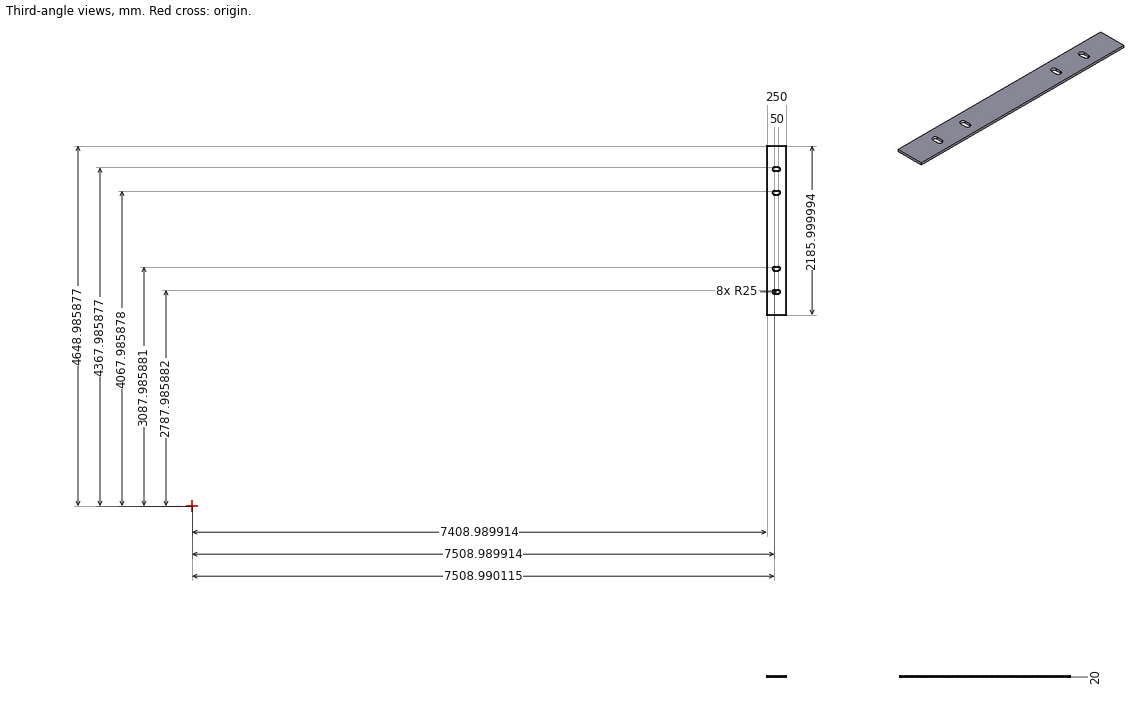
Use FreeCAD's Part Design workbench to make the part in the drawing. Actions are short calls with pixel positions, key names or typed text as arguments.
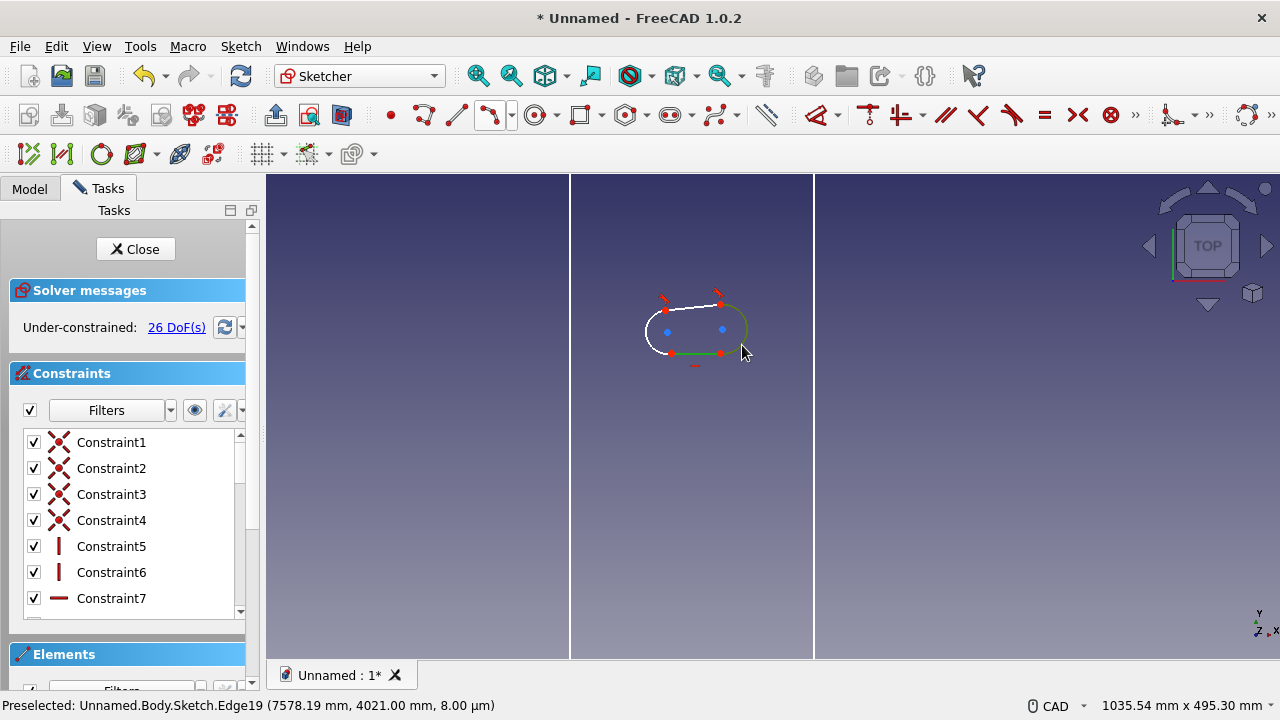
key(t)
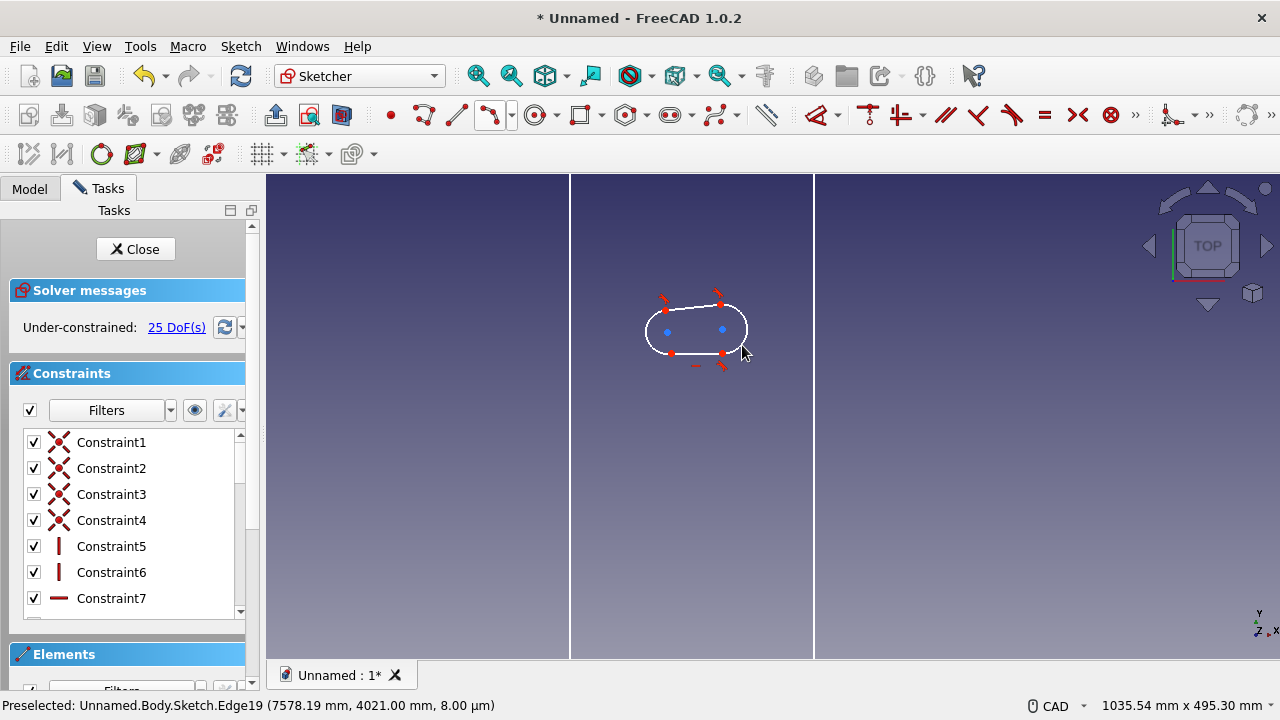
click(707, 354)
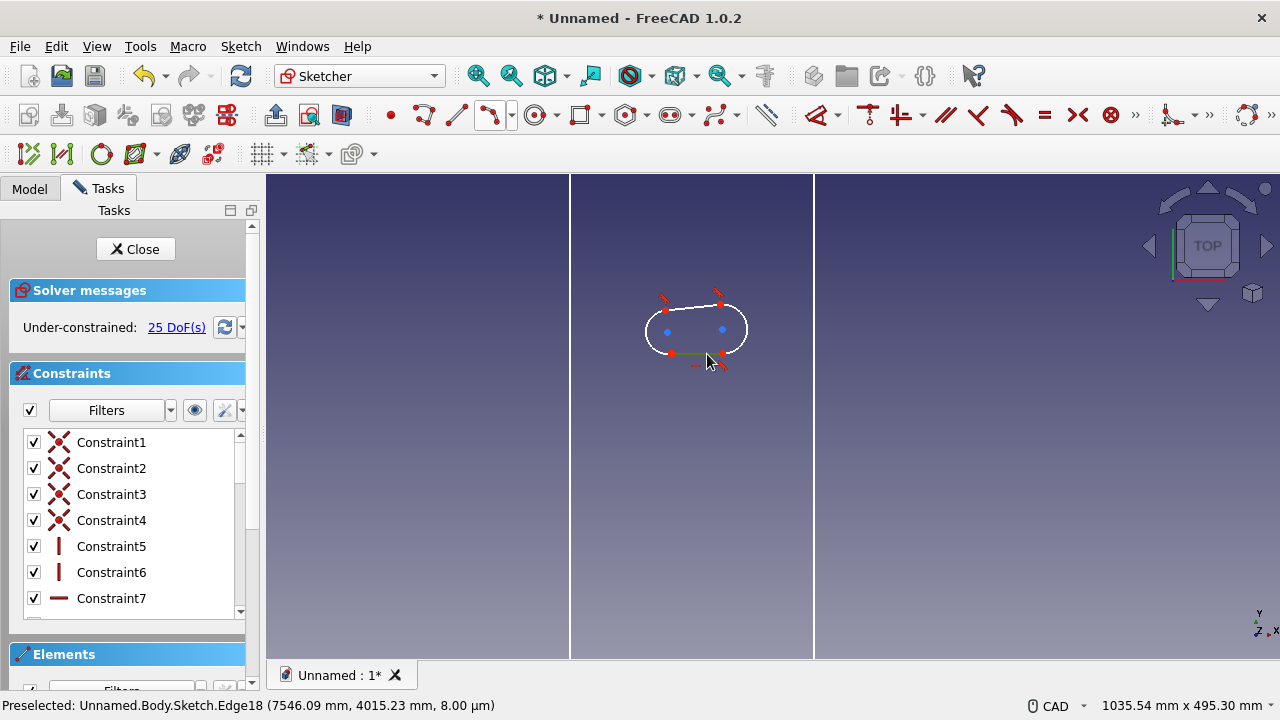
click(649, 322)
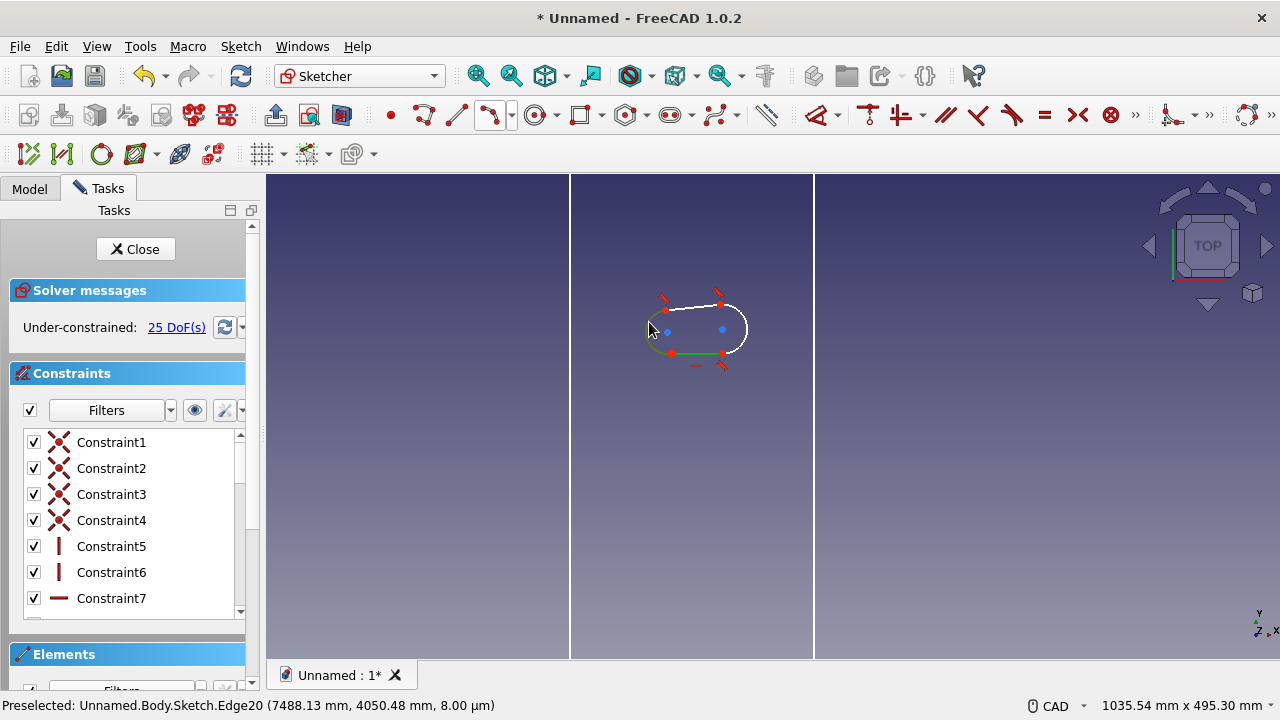
click(1012, 116)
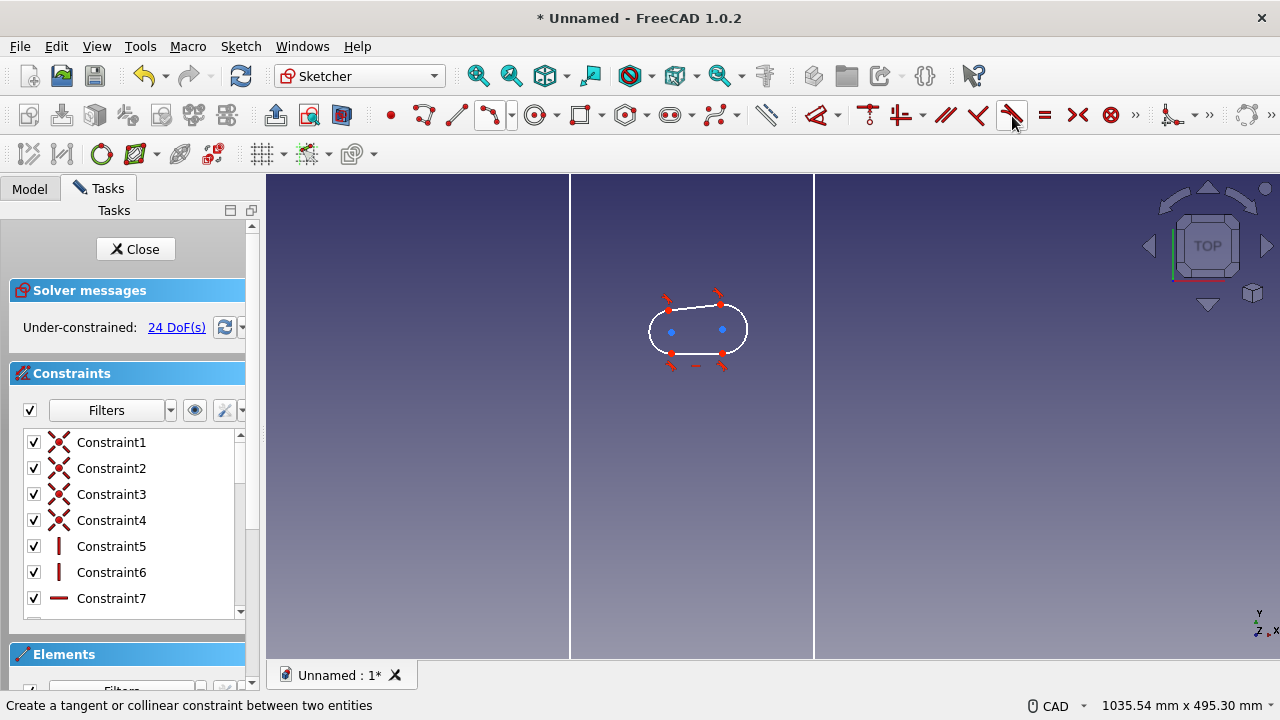
scroll(706, 356, down, 10)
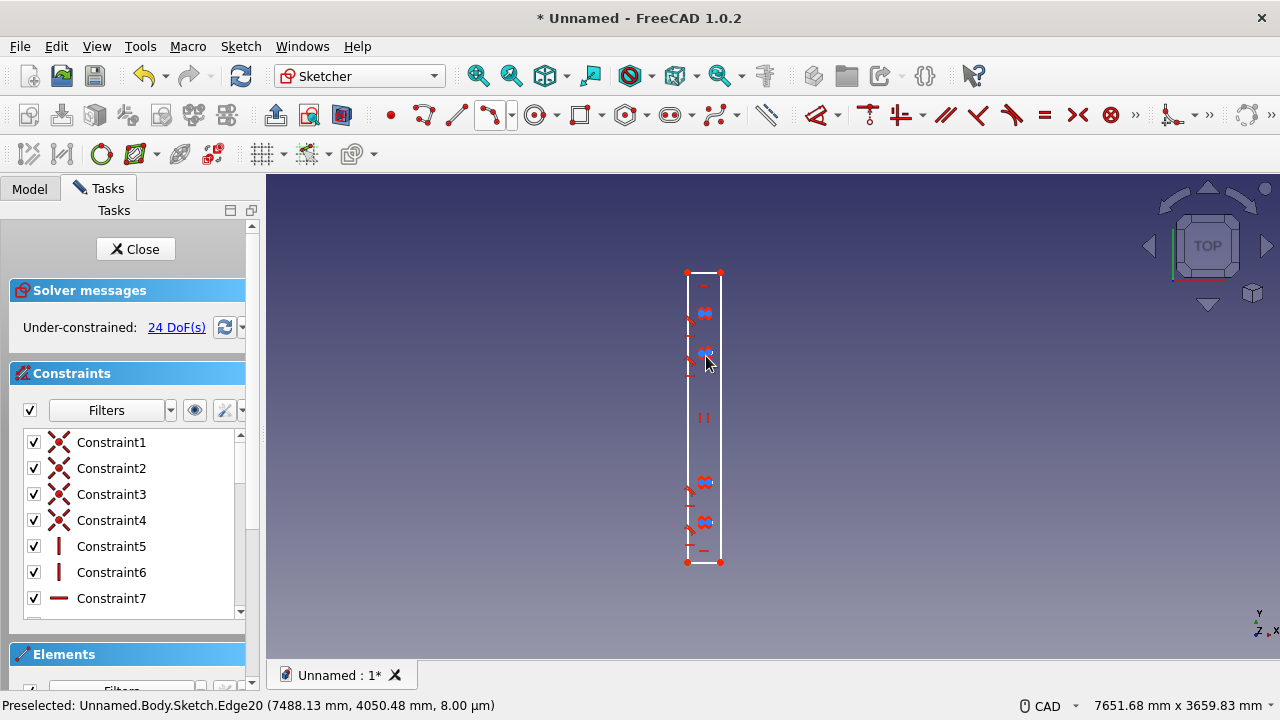
scroll(704, 520, up, 10)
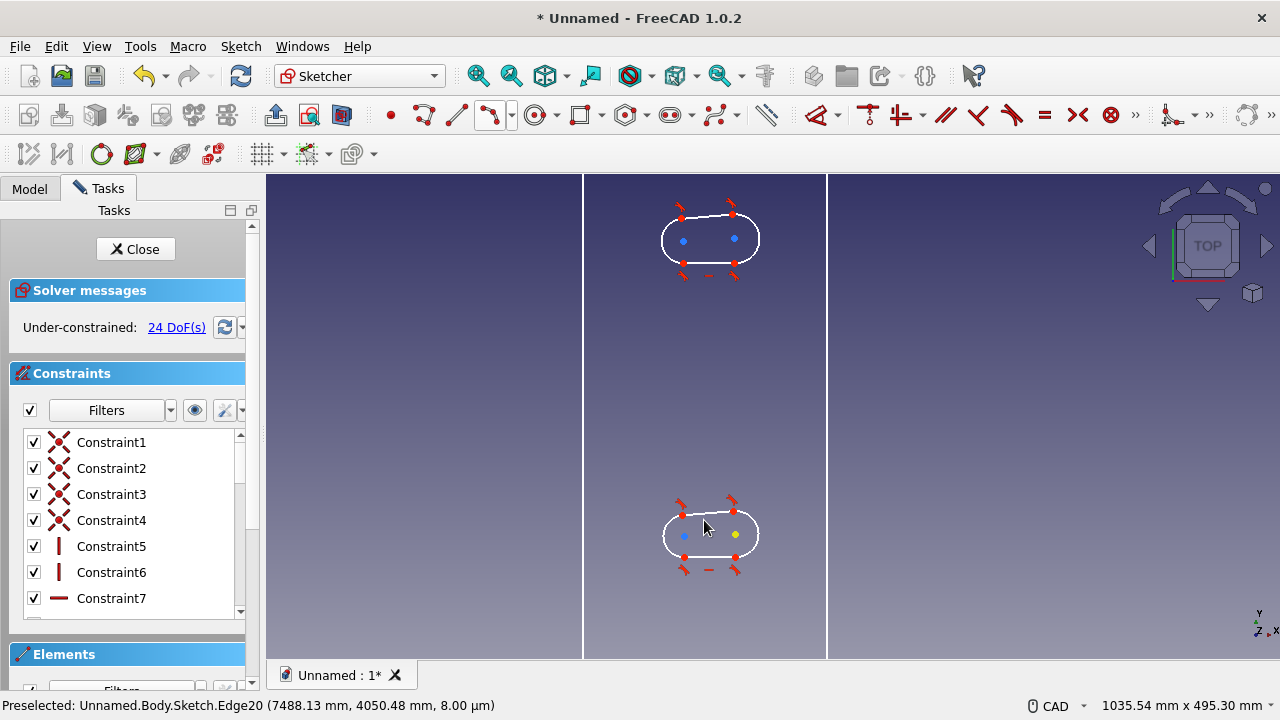
click(698, 514)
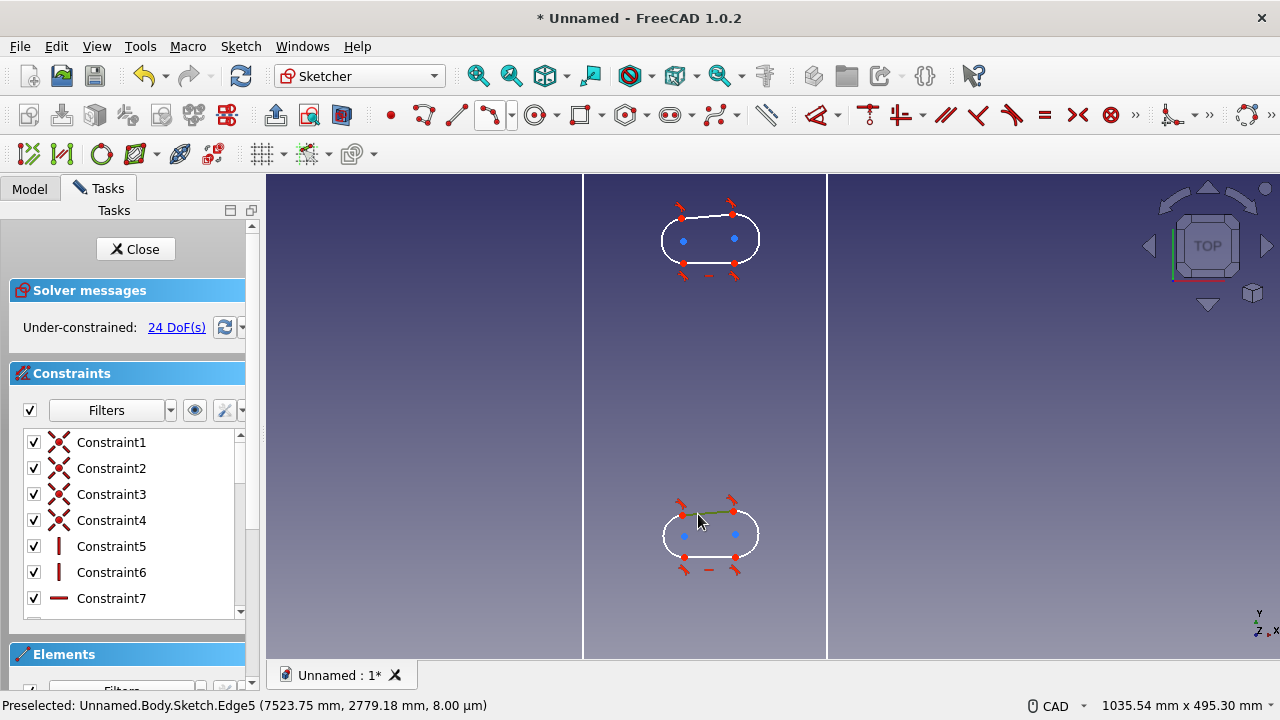
key(h)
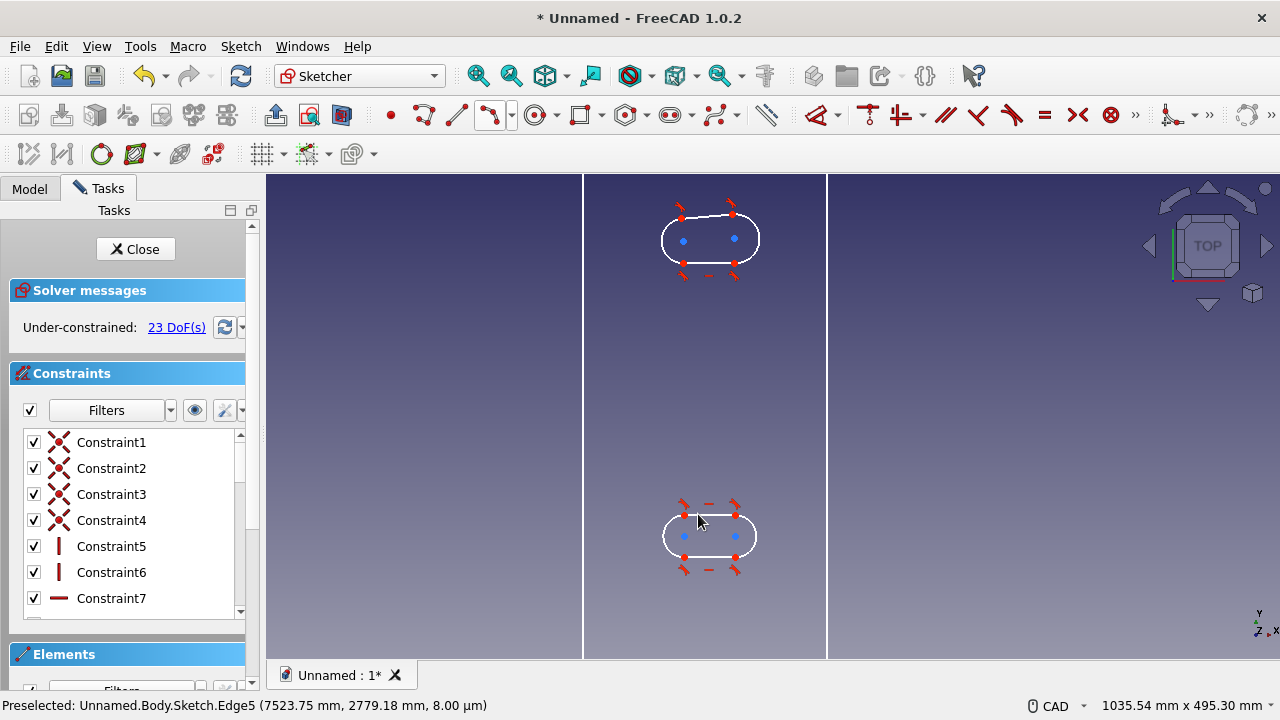
click(697, 218)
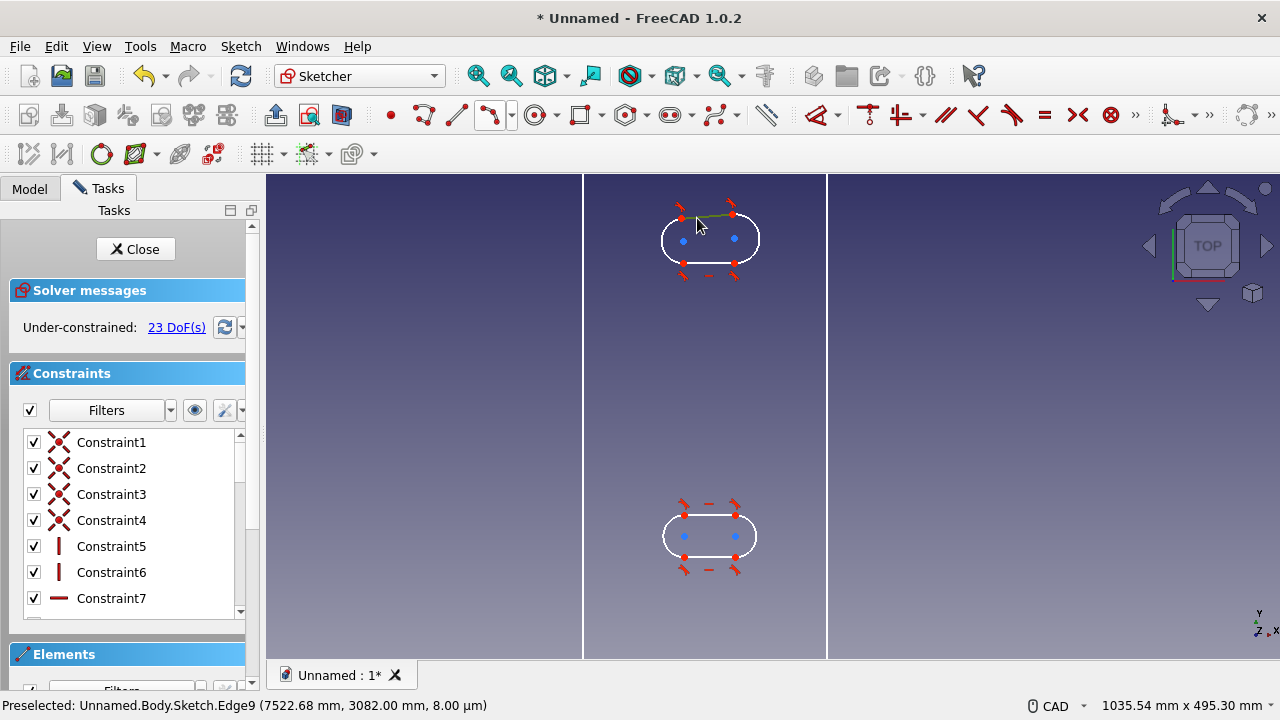
key(h)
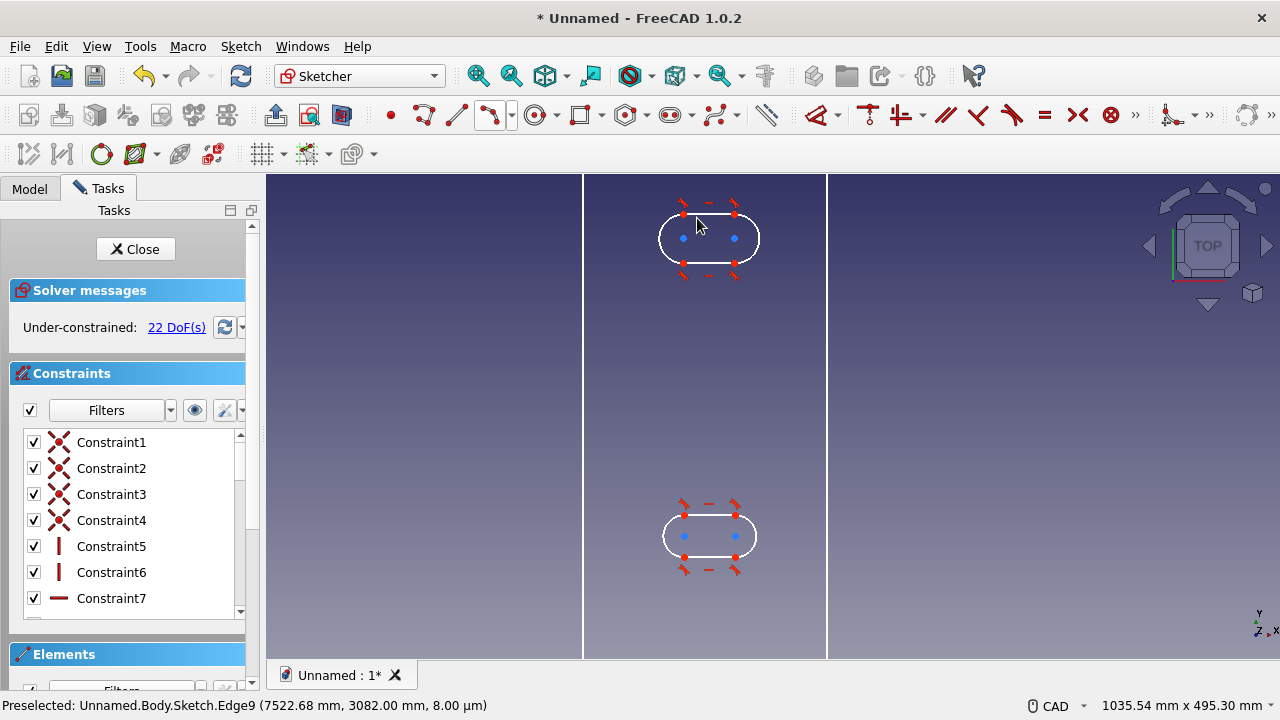
scroll(704, 520, down, 10)